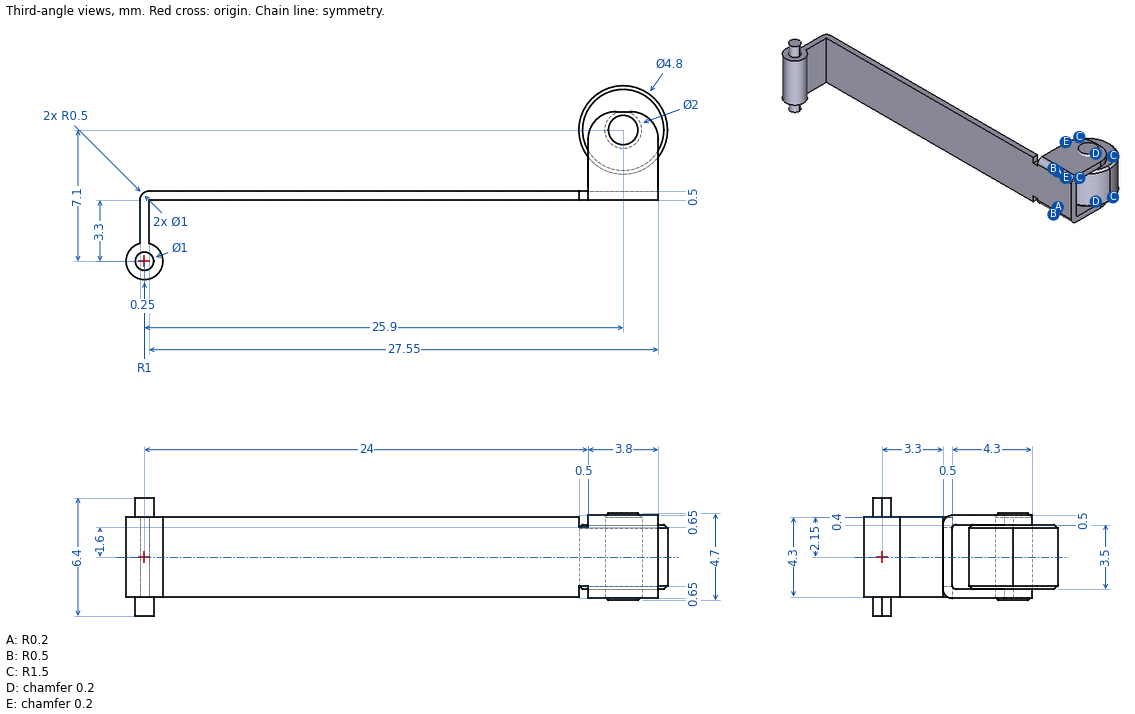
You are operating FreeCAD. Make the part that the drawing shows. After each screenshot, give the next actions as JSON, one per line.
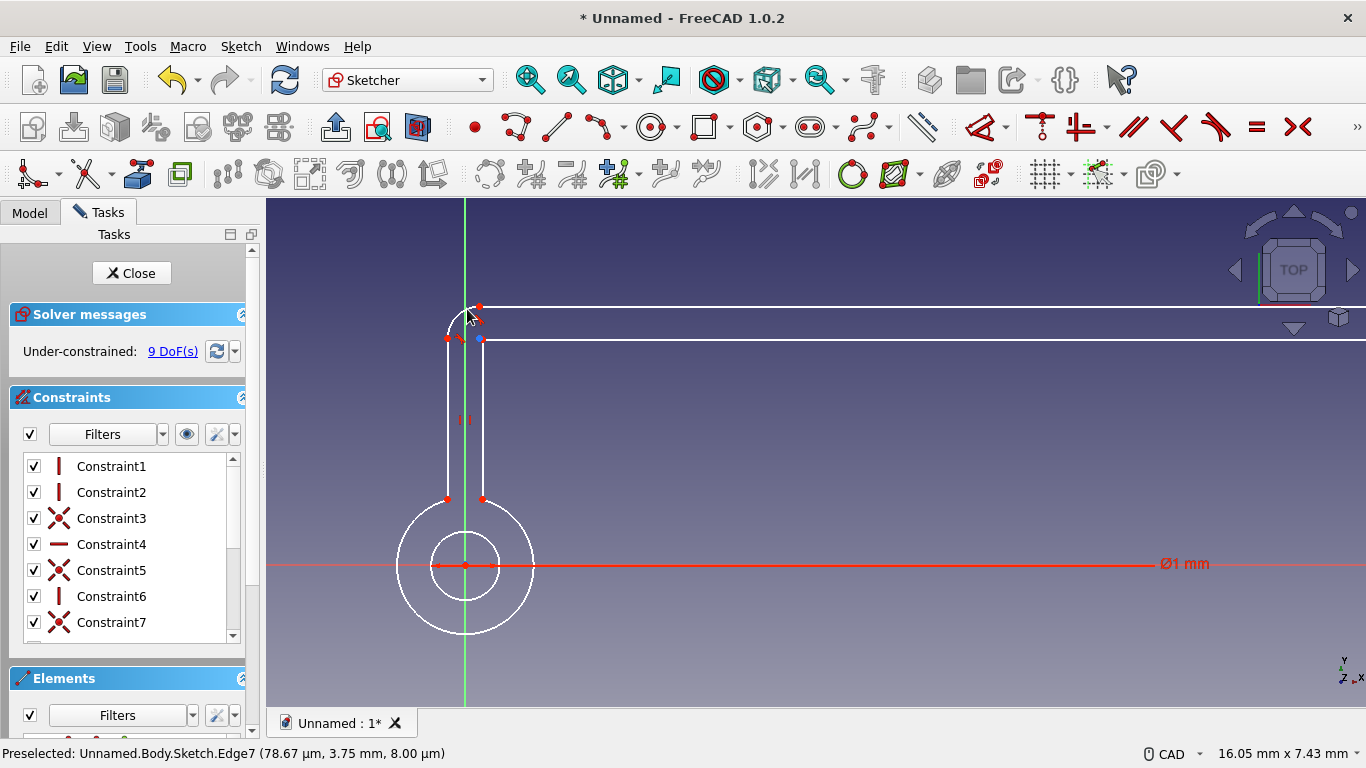
{"action": "scroll", "coordinate": [465, 565], "scroll_direction": "up", "scroll_amount": 2}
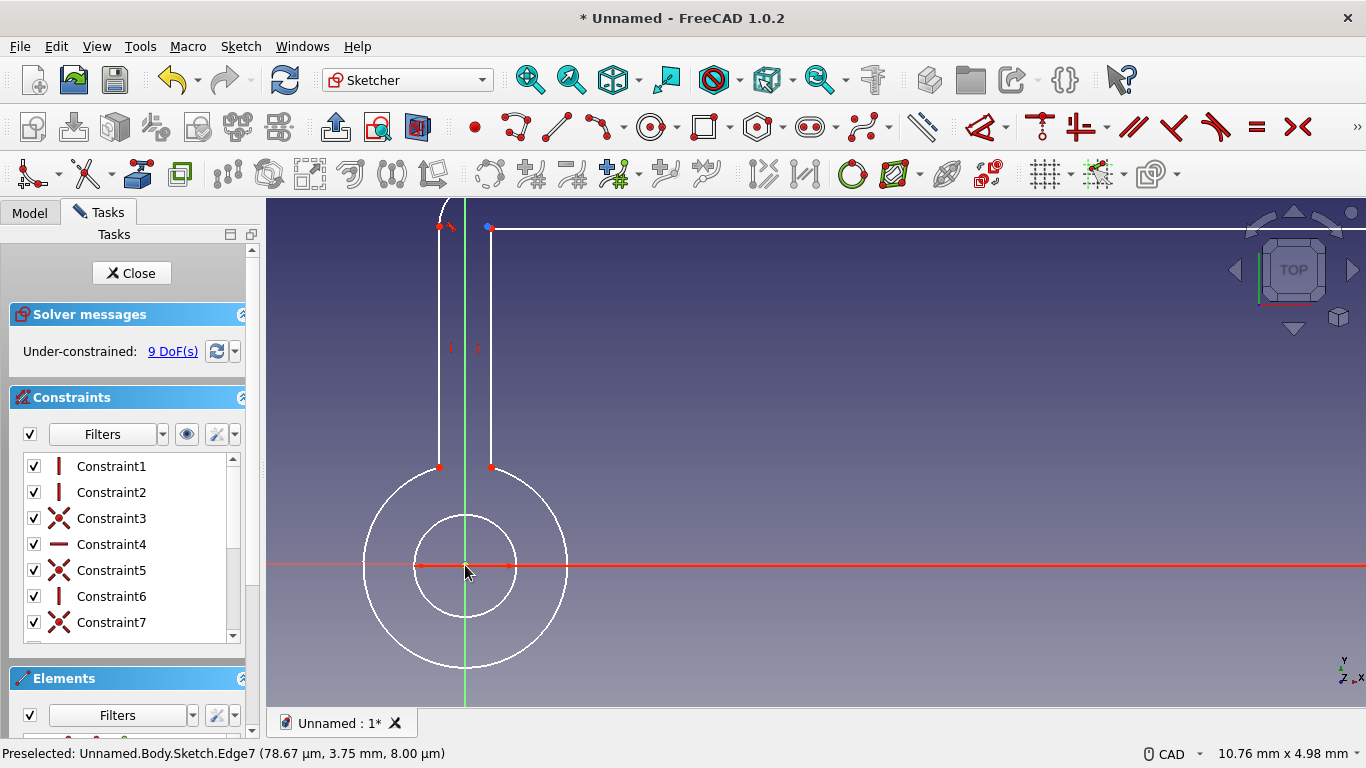
{"action": "left_click_drag", "start_coordinate": [455, 554], "coordinate": [475, 576]}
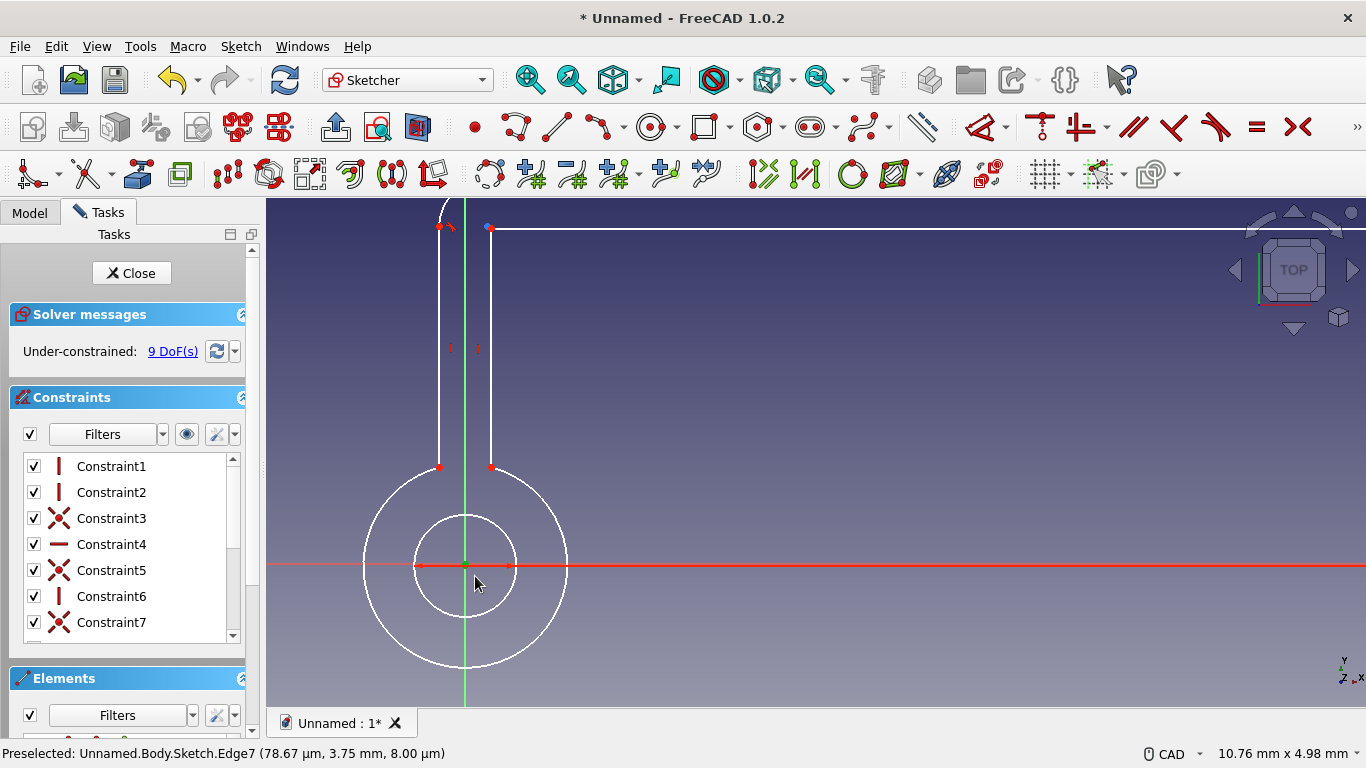
{"action": "key", "text": "c"}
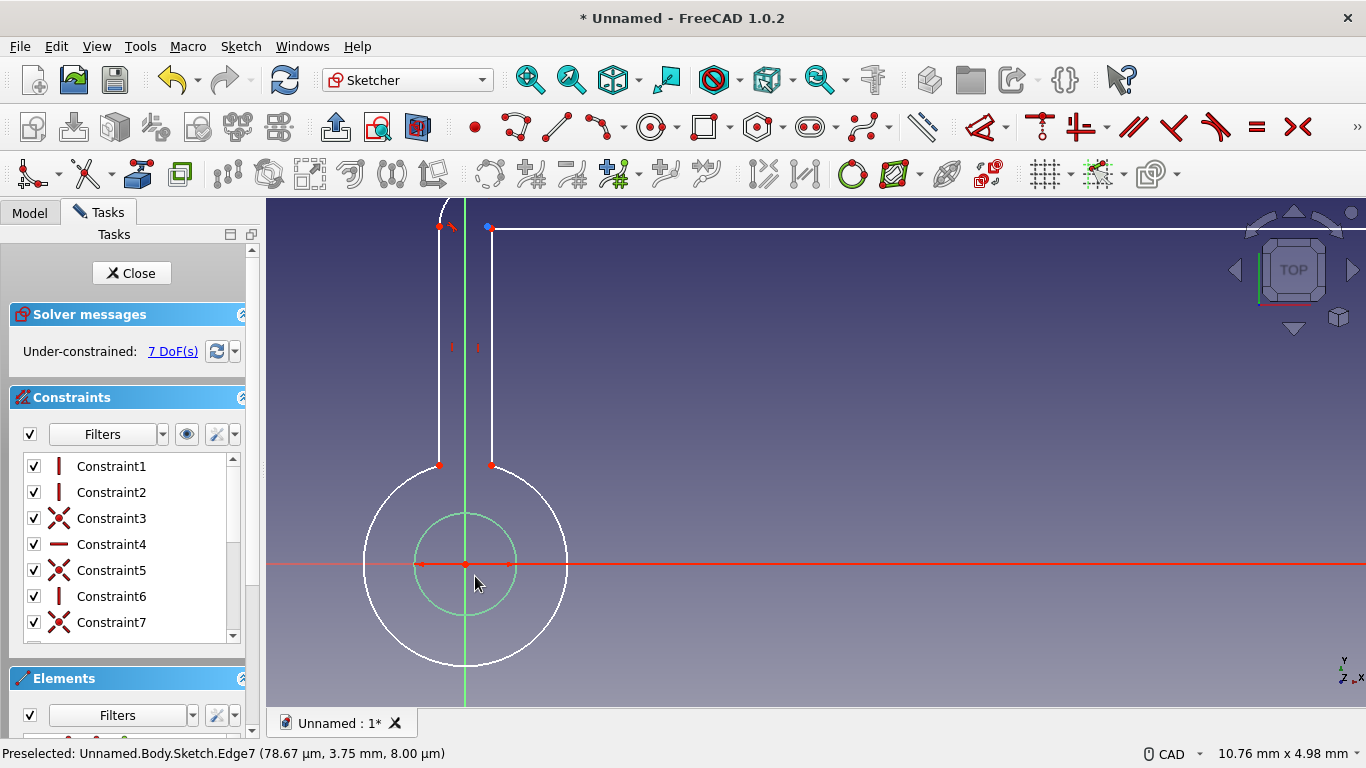
{"action": "left_click", "coordinate": [980, 128]}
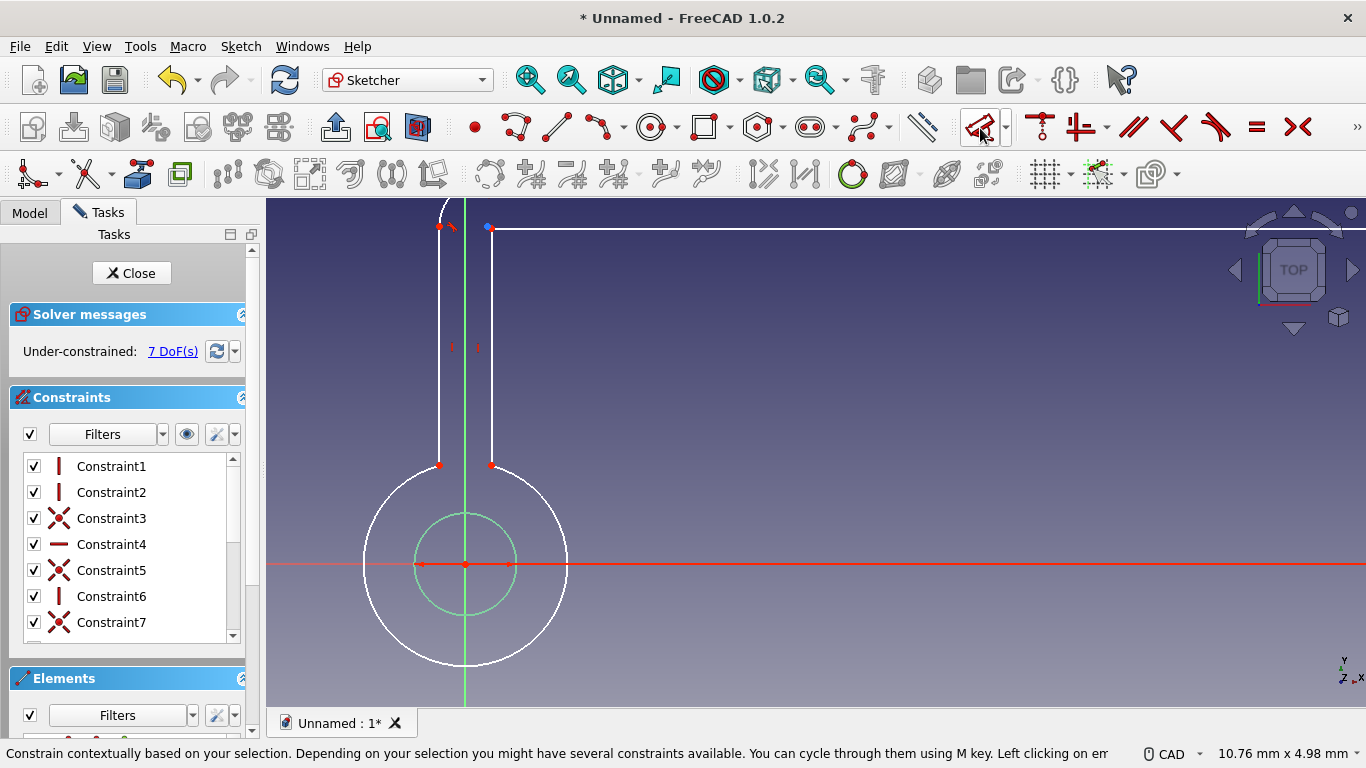
{"action": "left_click", "coordinate": [372, 606]}
{"action": "left_click", "coordinate": [343, 619]}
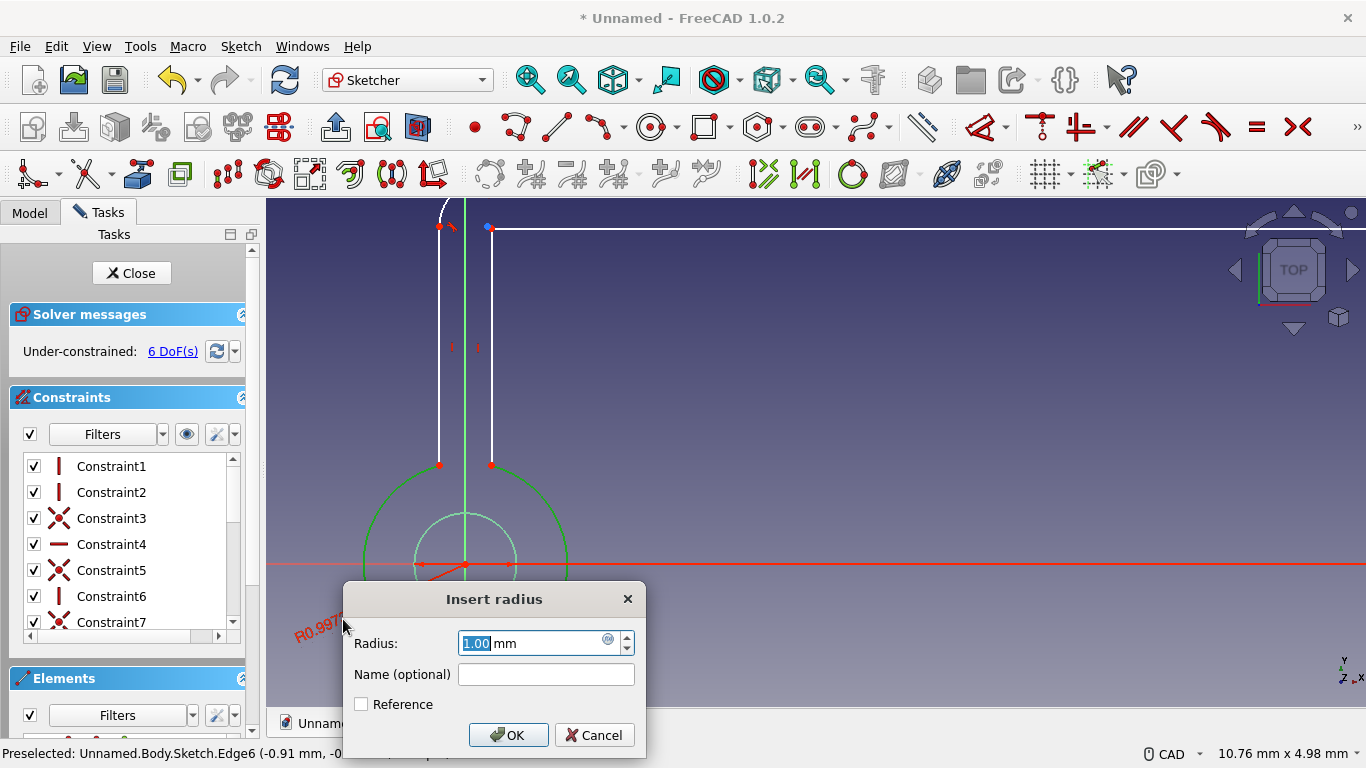
{"action": "type", "text": "1"}
{"action": "key", "text": "Return"}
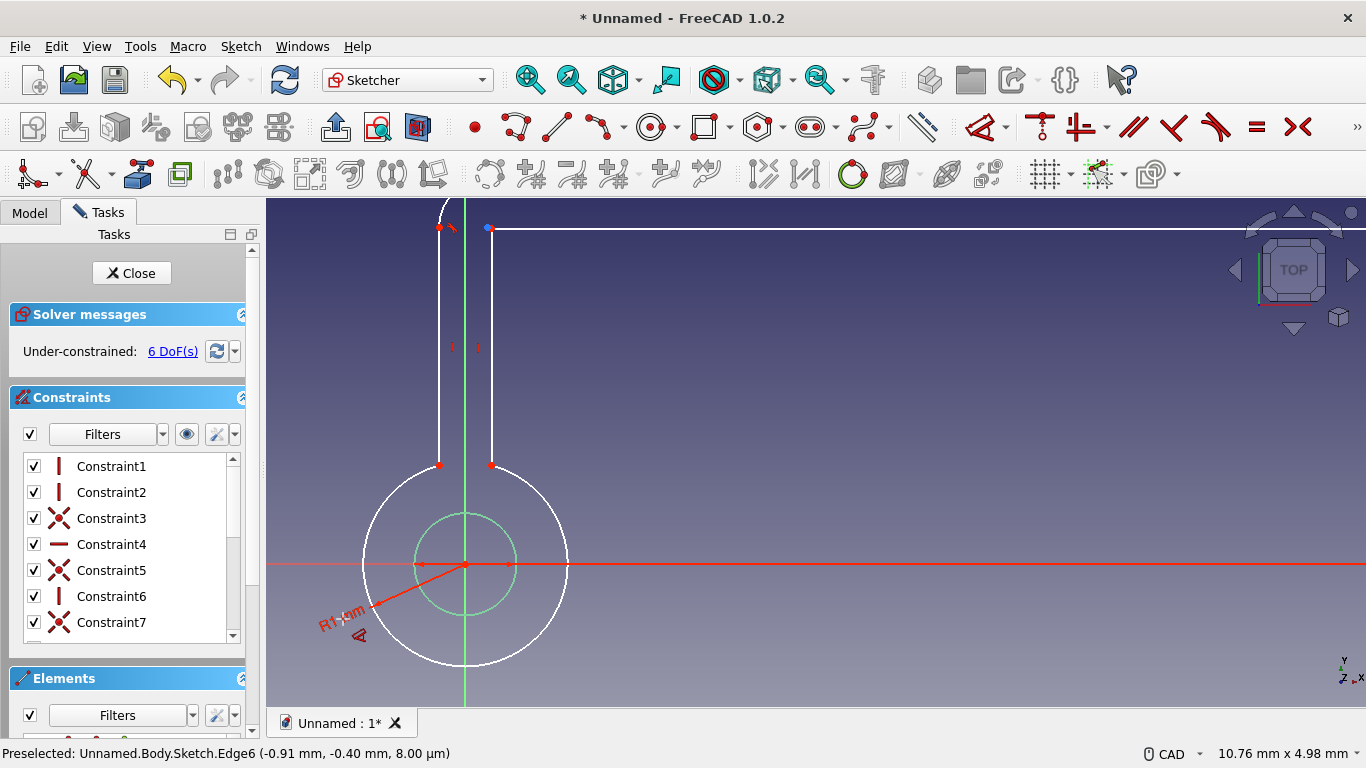
{"action": "scroll", "coordinate": [466, 460], "scroll_direction": "down", "scroll_amount": 8}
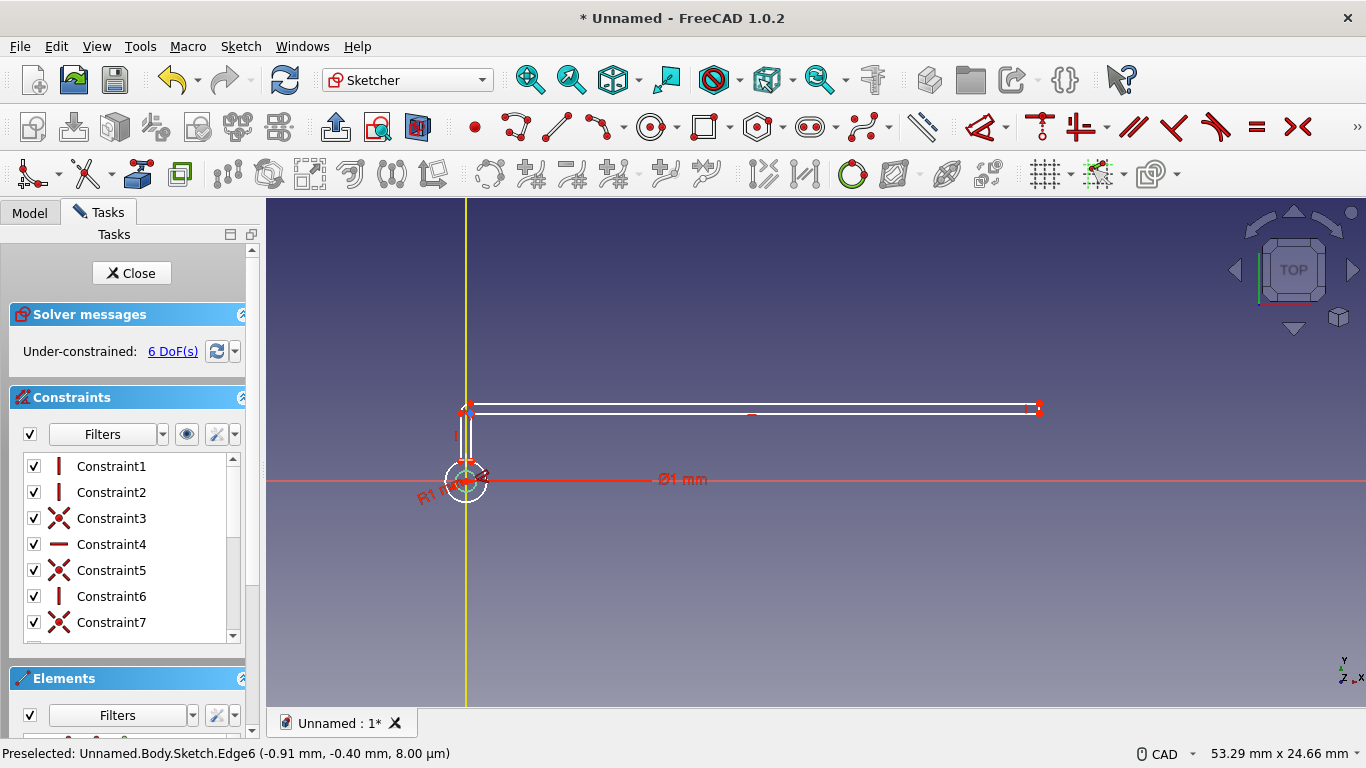
{"action": "scroll", "coordinate": [466, 405], "scroll_direction": "up", "scroll_amount": 7}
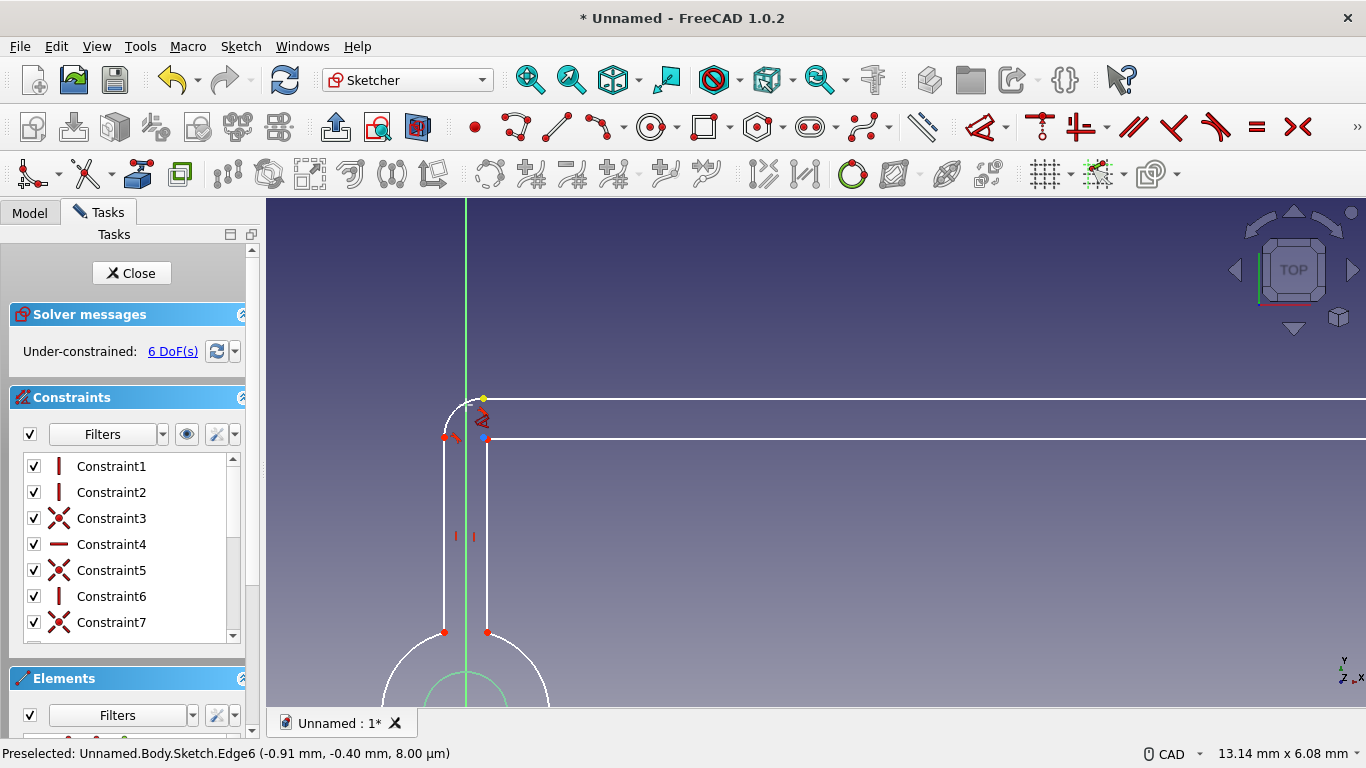
{"action": "left_click", "coordinate": [466, 403]}
{"action": "left_click", "coordinate": [452, 374]}